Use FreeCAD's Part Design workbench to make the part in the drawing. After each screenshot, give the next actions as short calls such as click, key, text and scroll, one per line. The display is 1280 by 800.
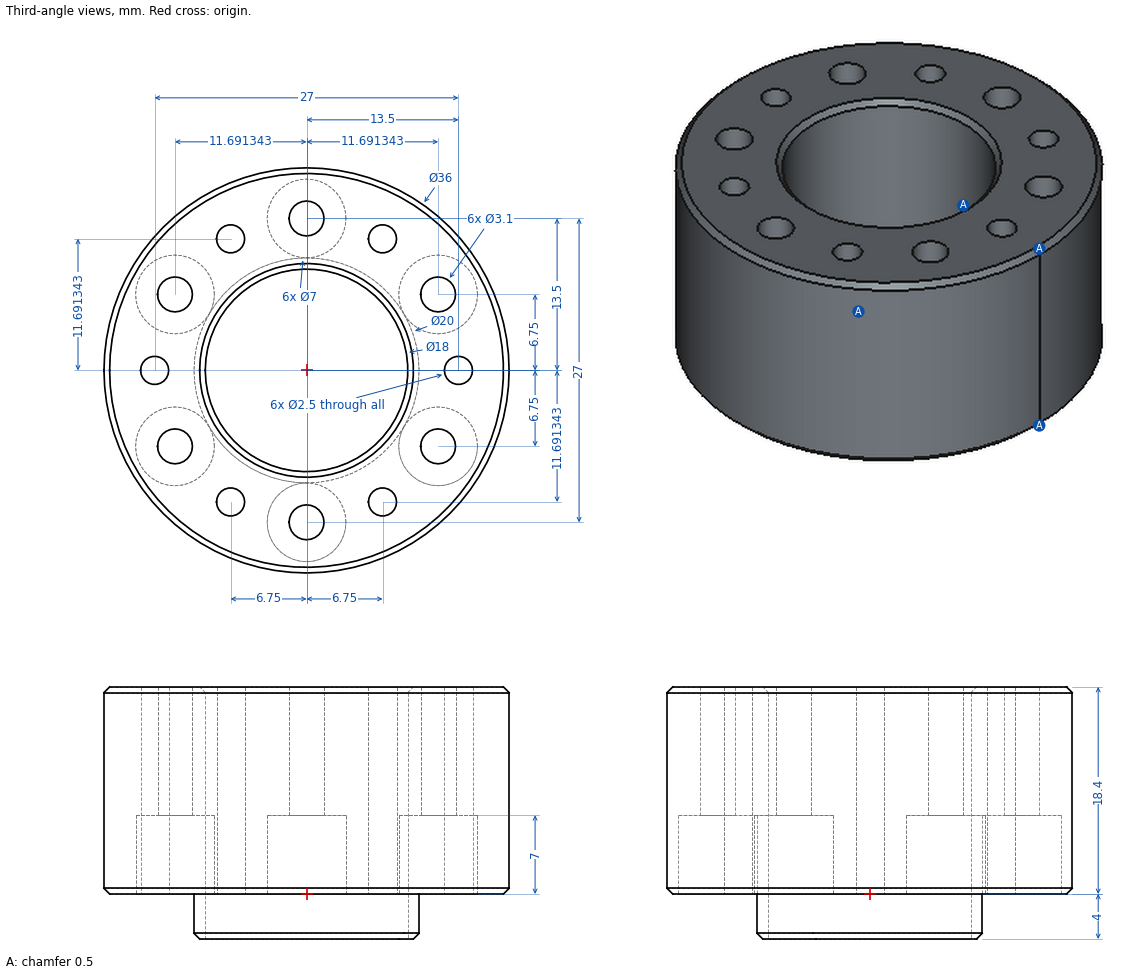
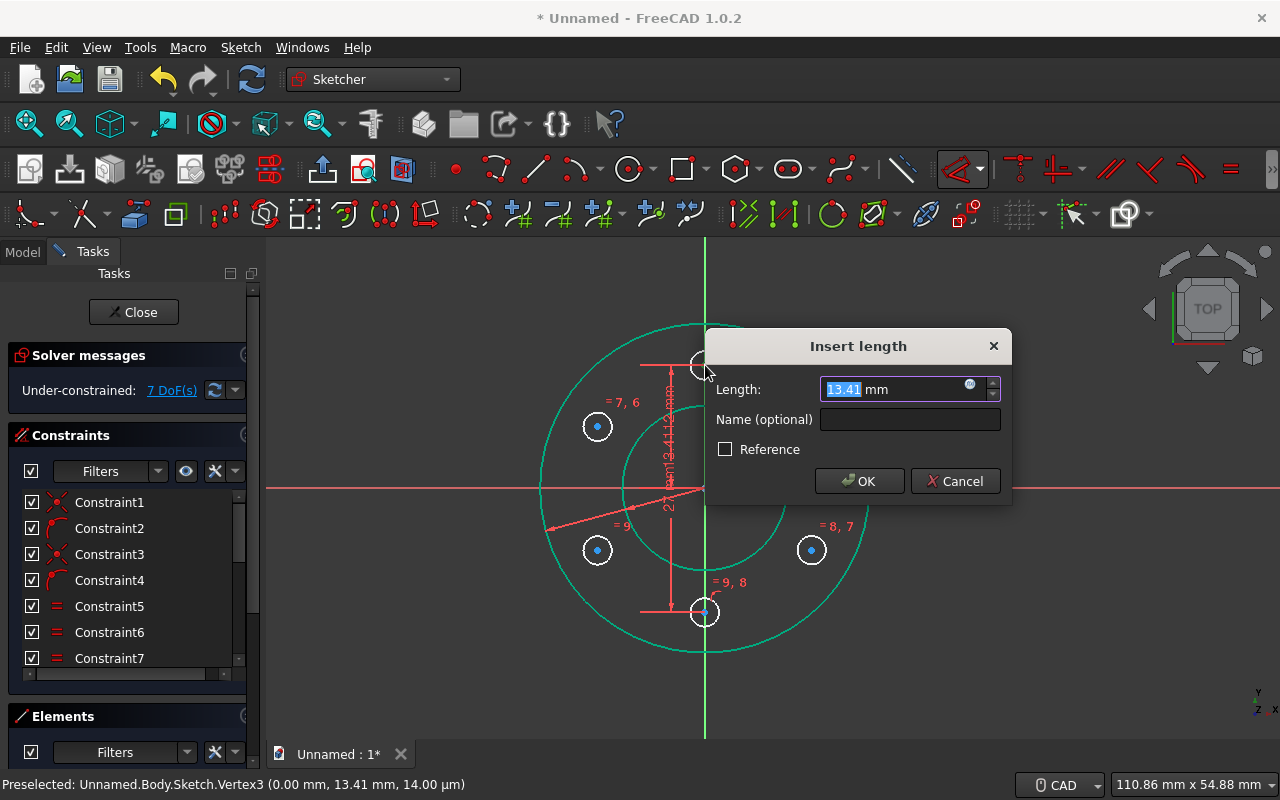
text(13.5)
key(Return)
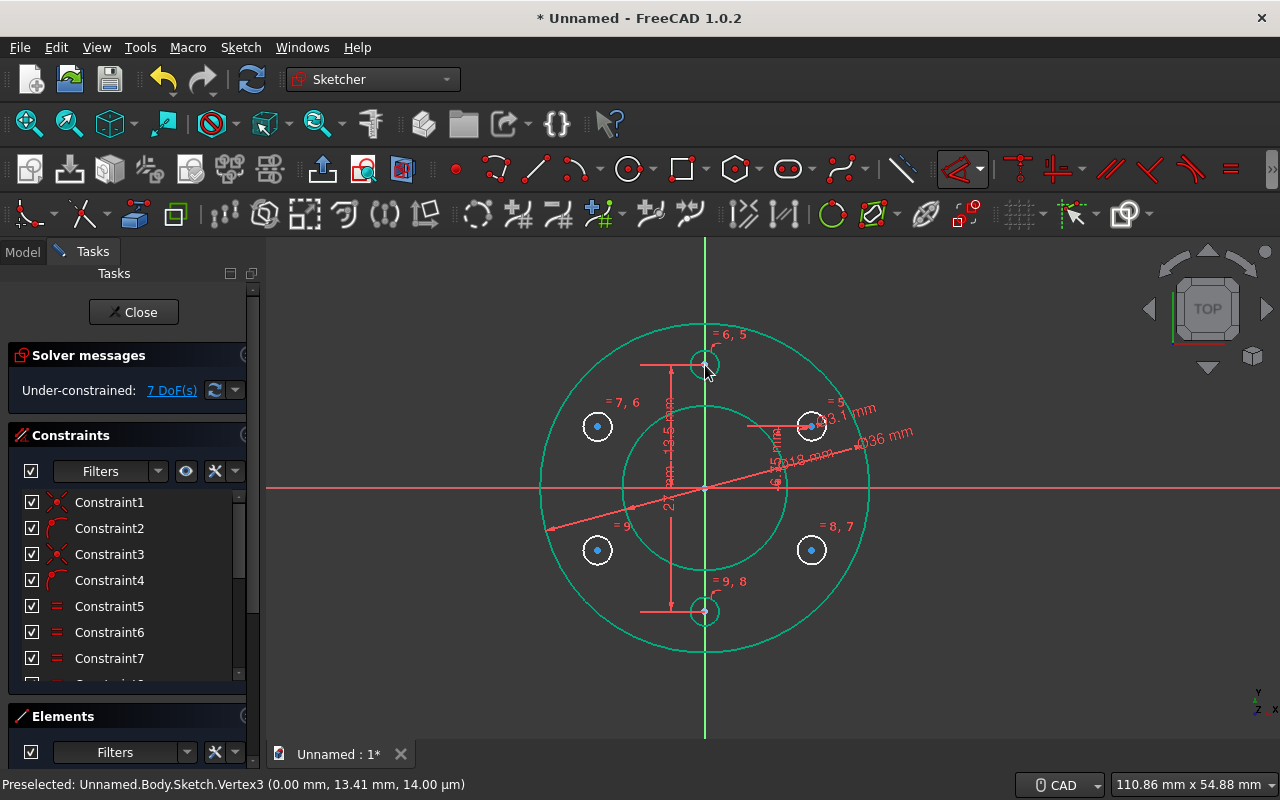
click(598, 427)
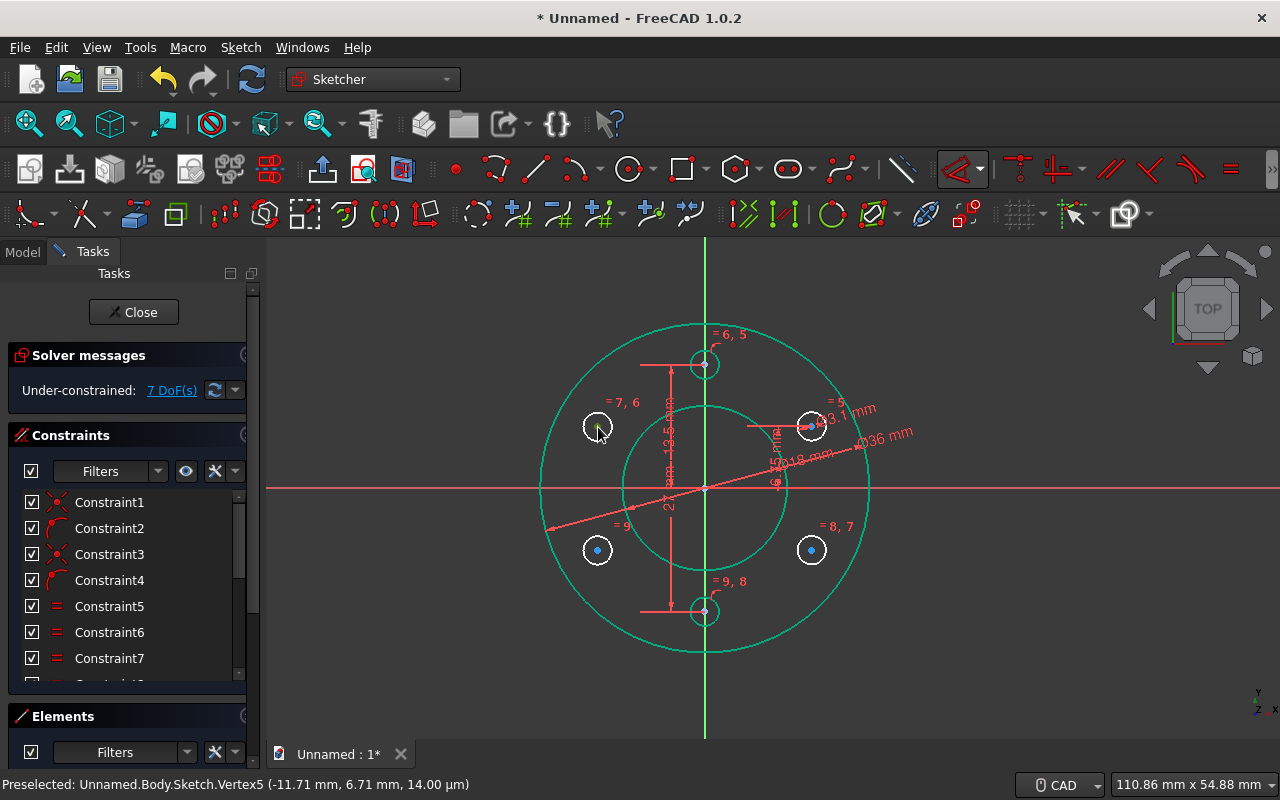
click(982, 170)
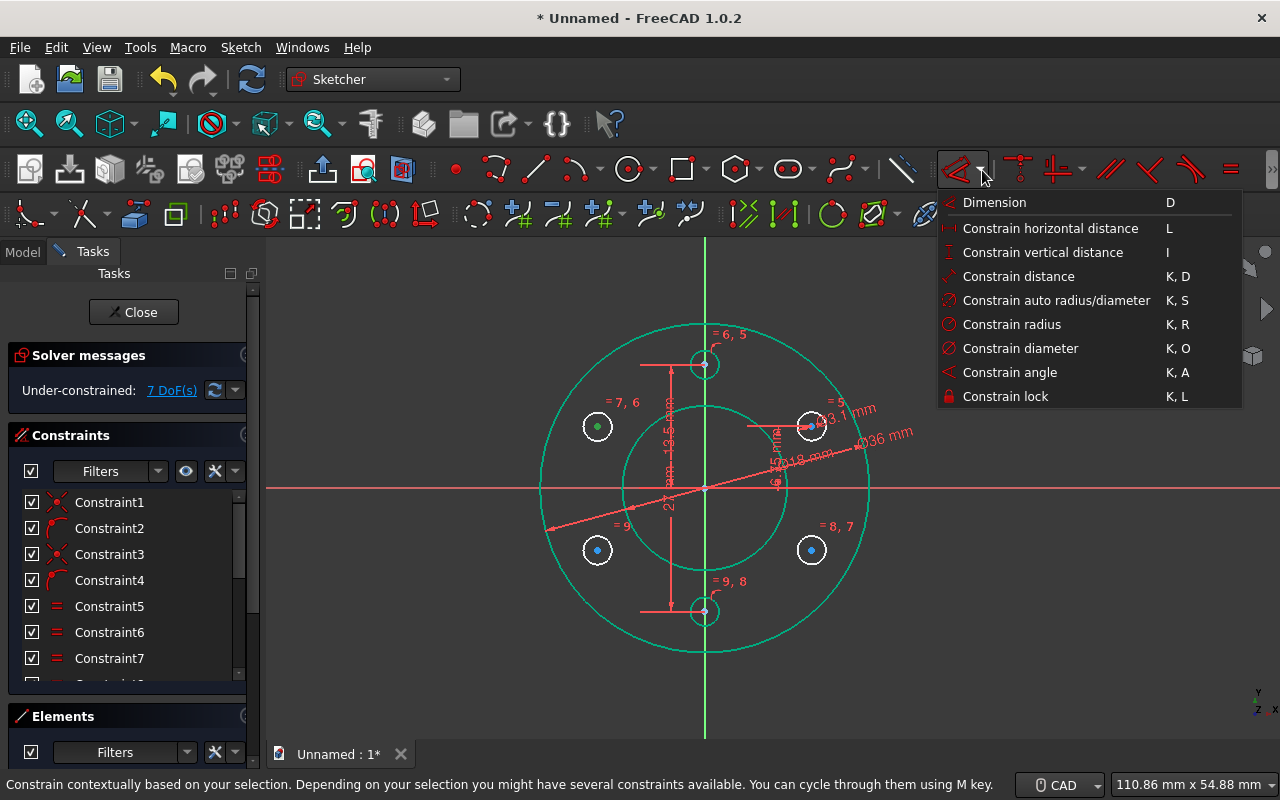
click(1090, 252)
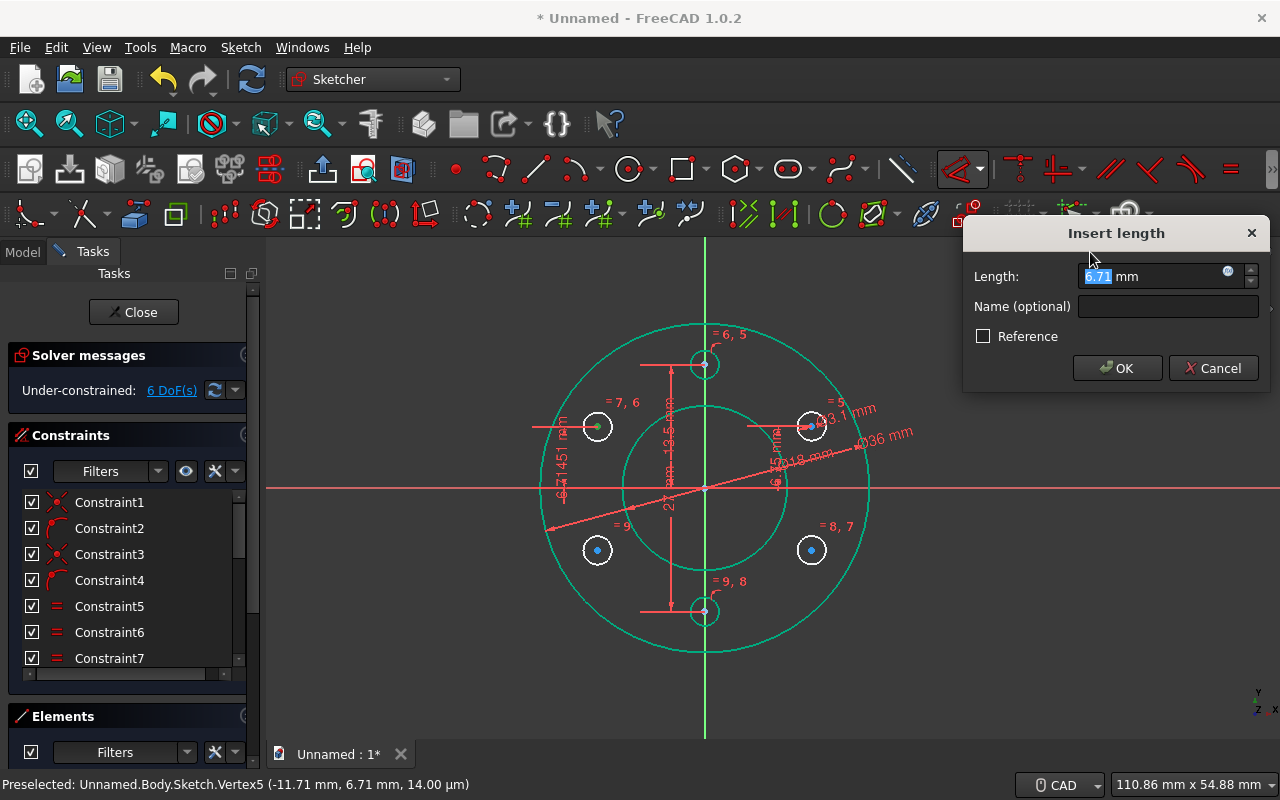
text(6.75)
key(Return)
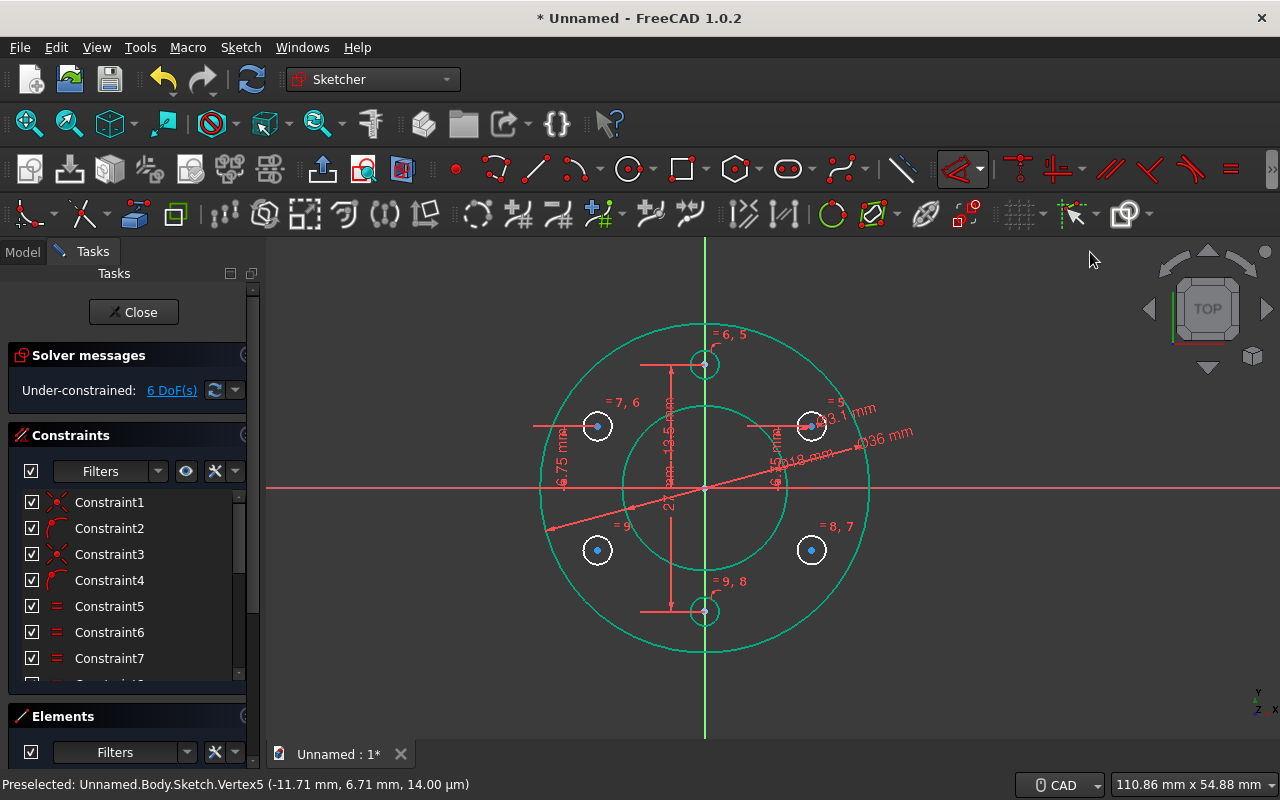
click(812, 550)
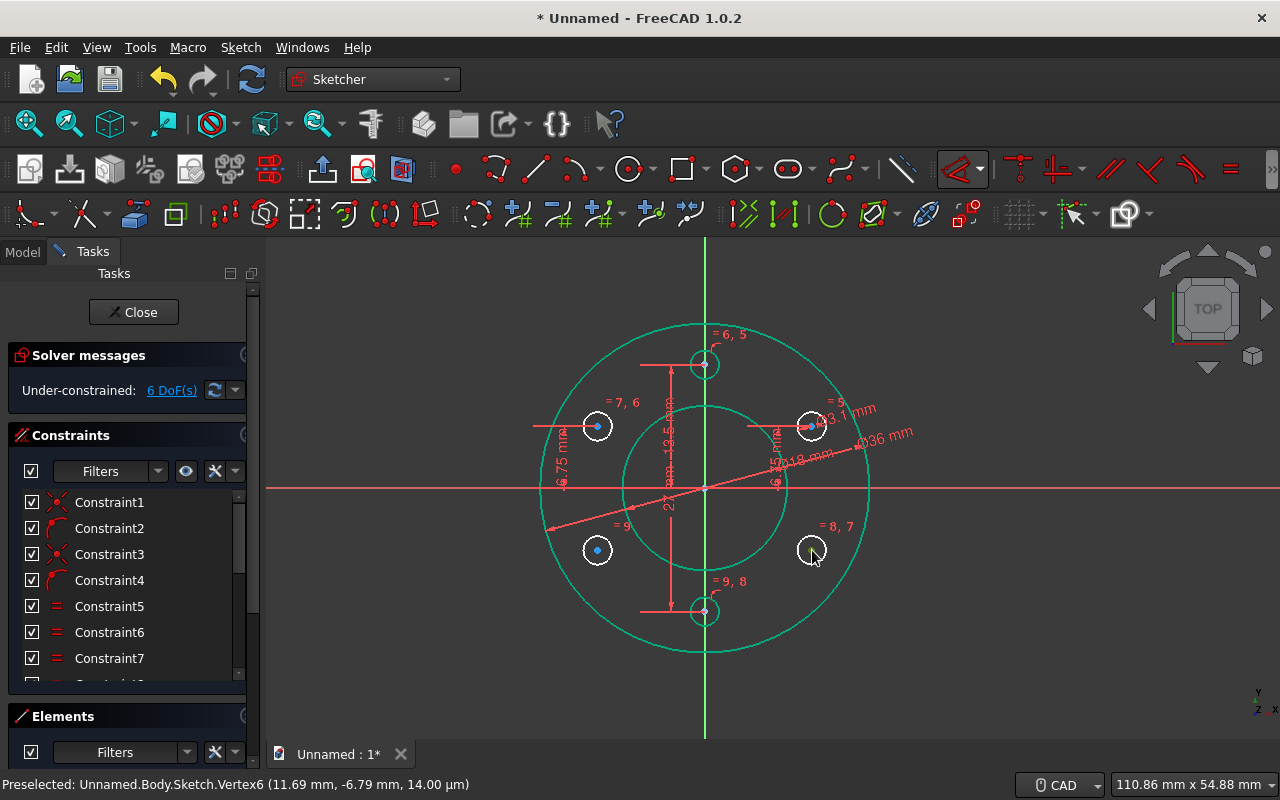
click(982, 170)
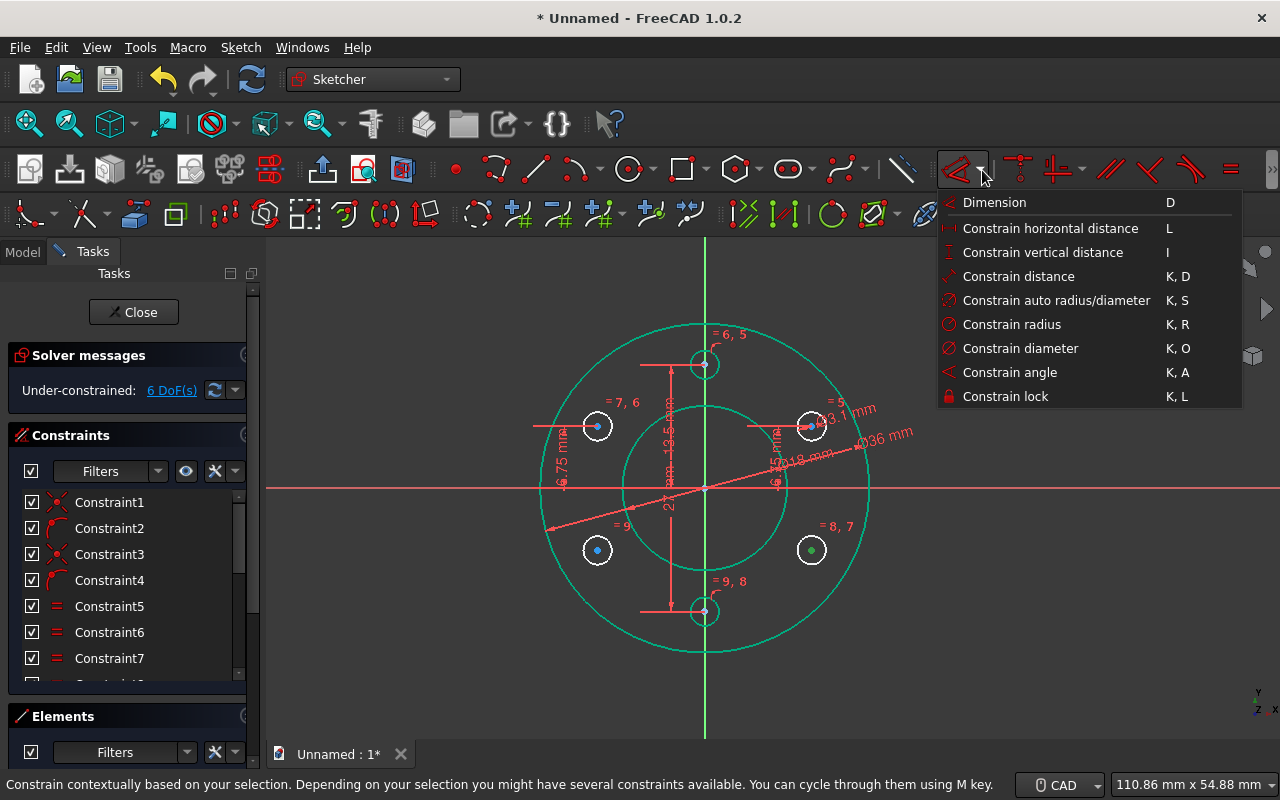
click(1090, 252)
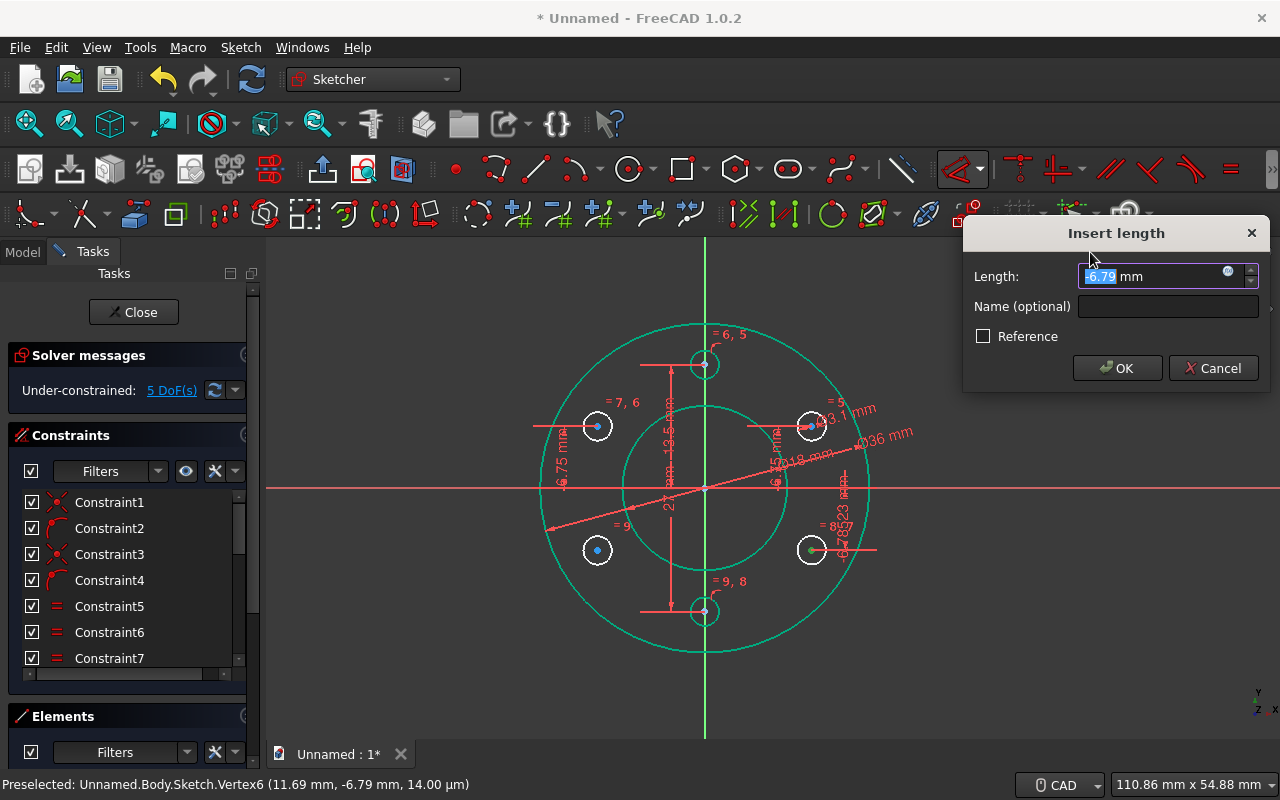
text(-6.75)
key(Return)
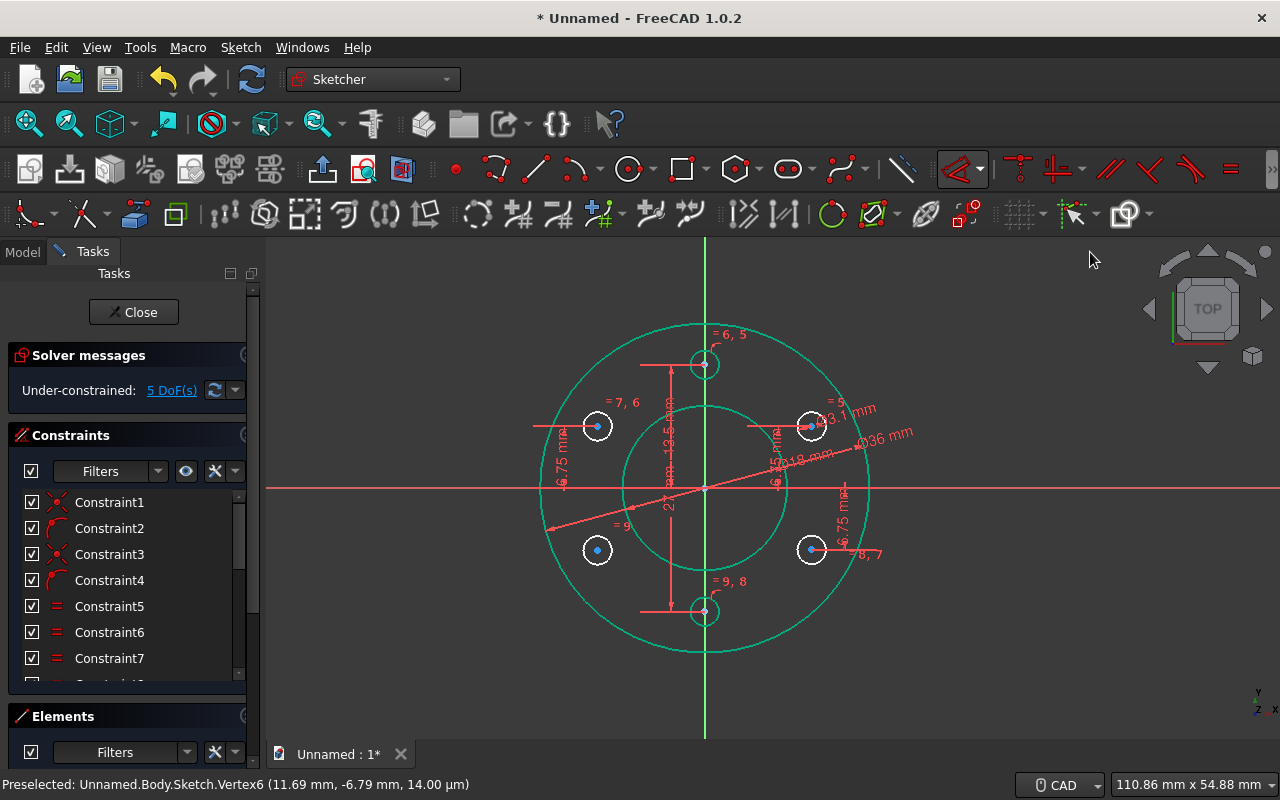
click(598, 550)